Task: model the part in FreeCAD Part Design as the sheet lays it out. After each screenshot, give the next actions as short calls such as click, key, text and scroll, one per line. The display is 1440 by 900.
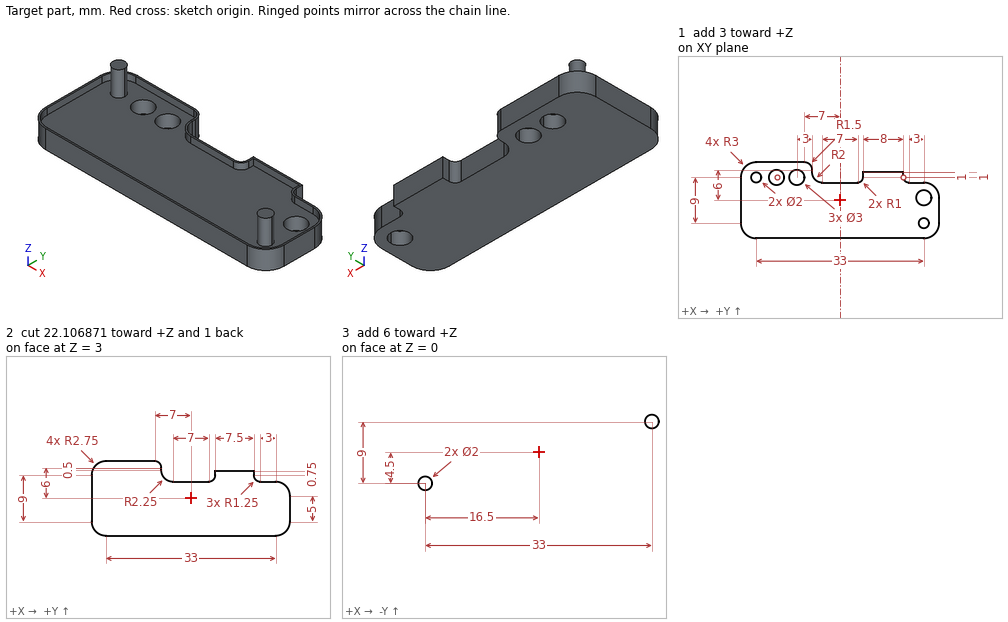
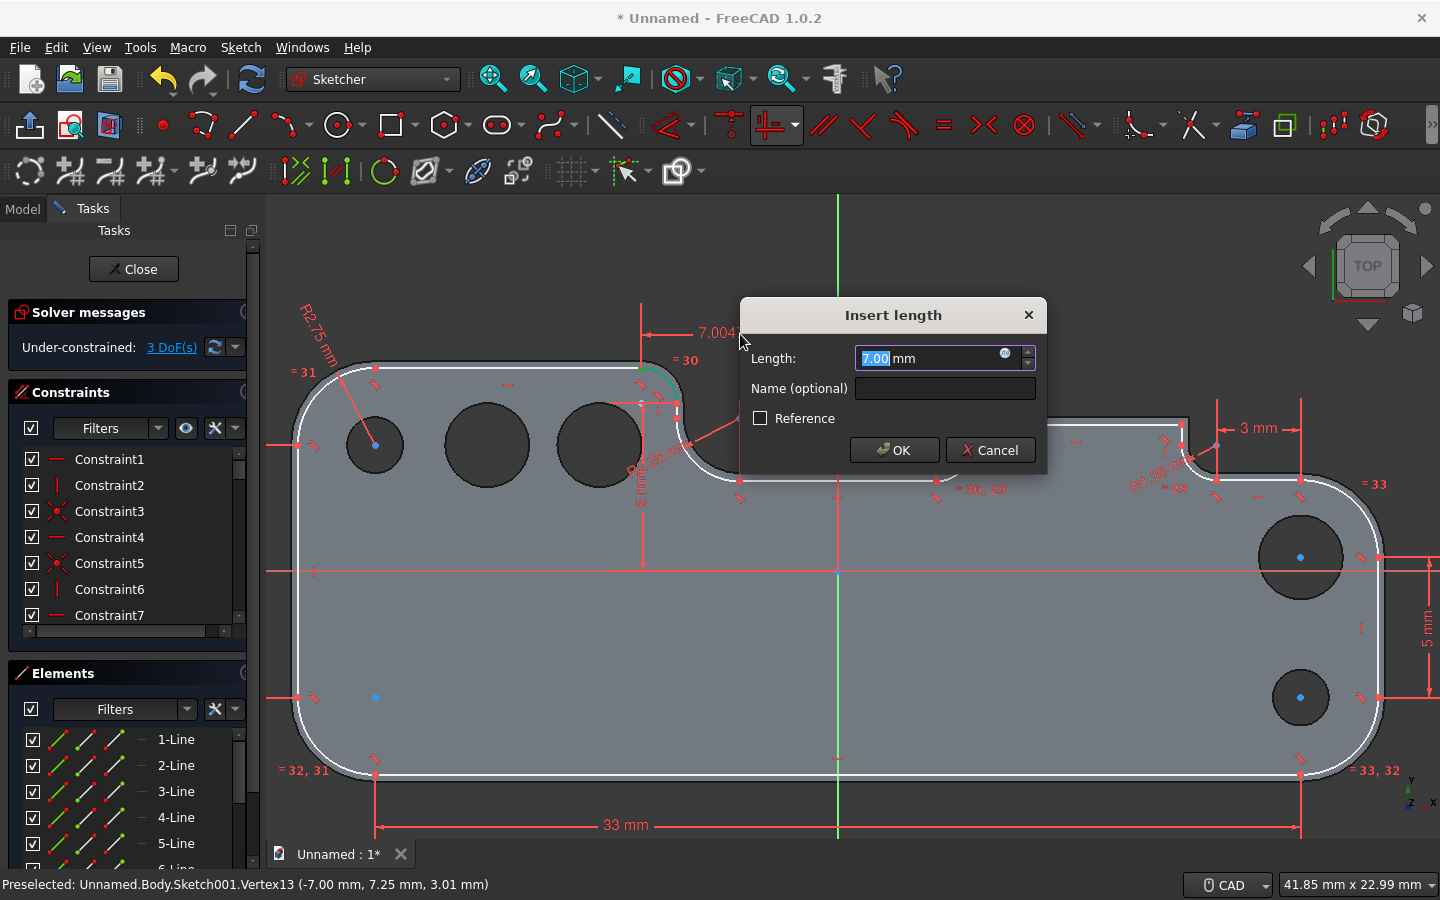
text(7)
key(Return)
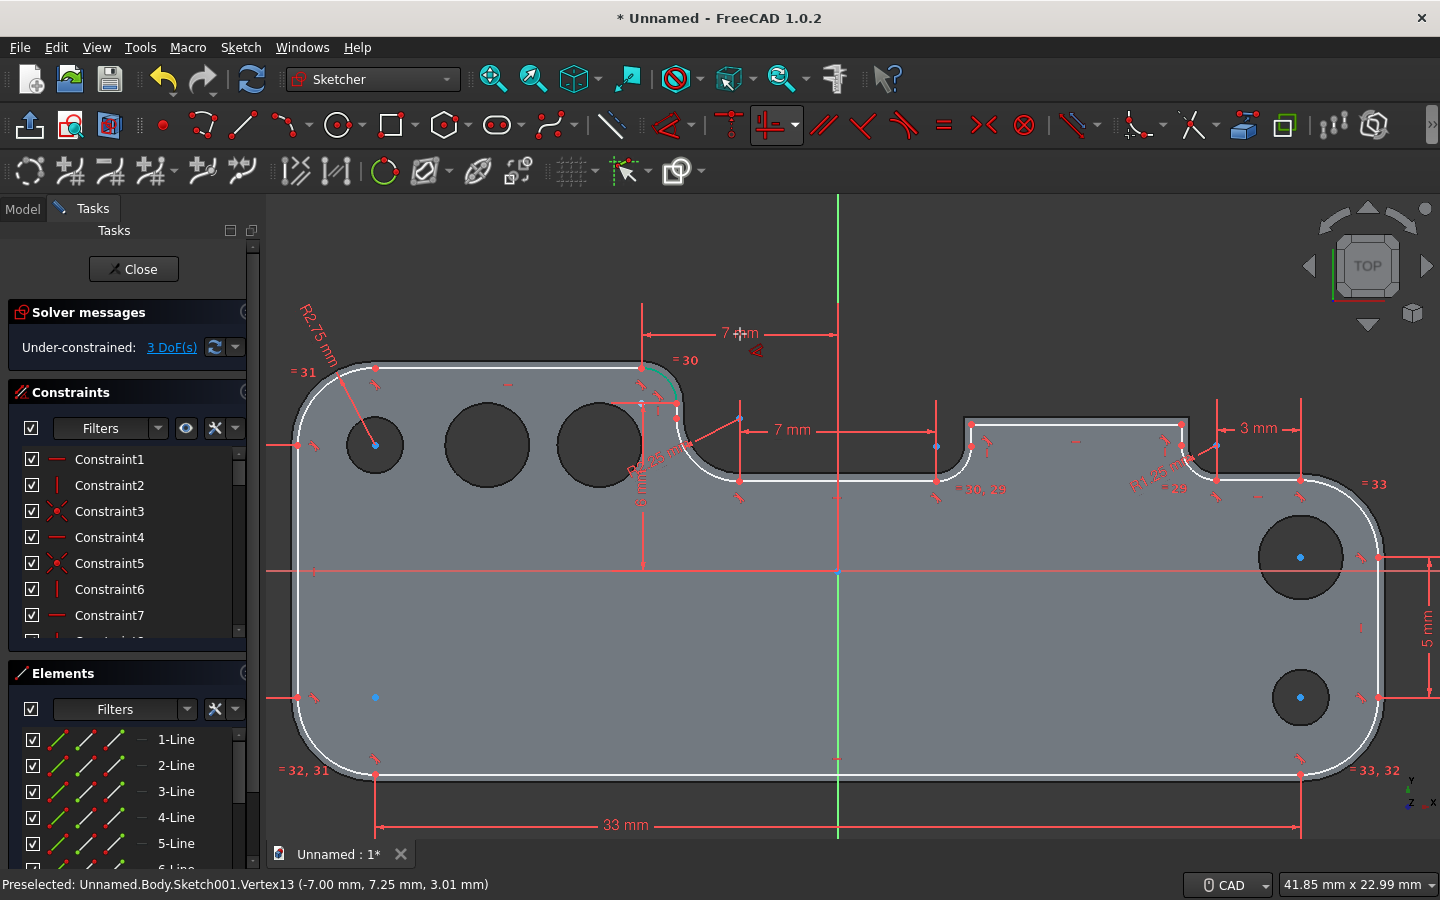
click(1119, 425)
click(1076, 391)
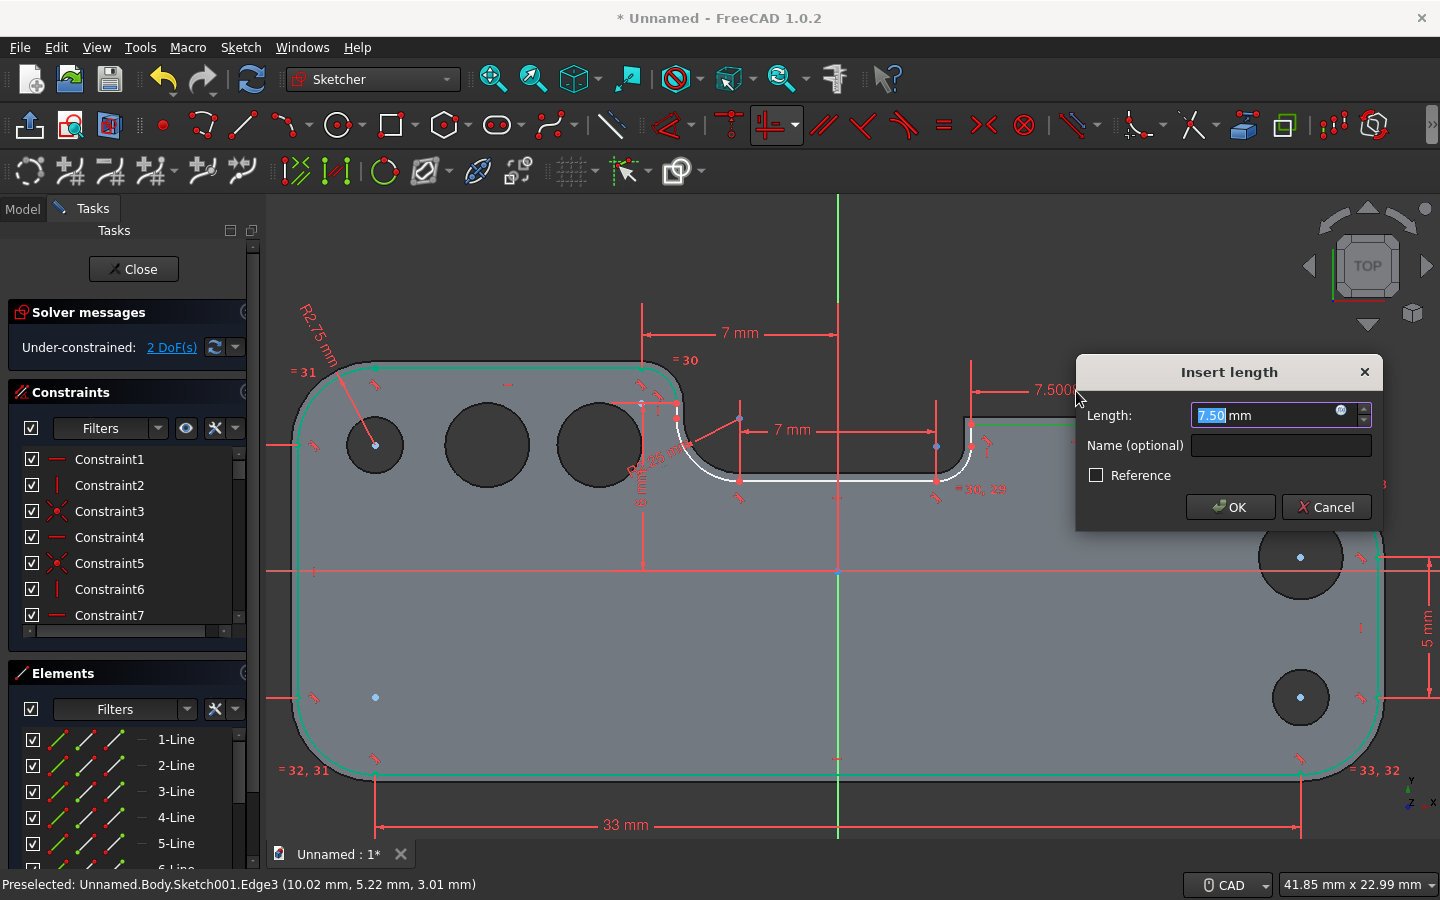
text(7.5)
key(Return)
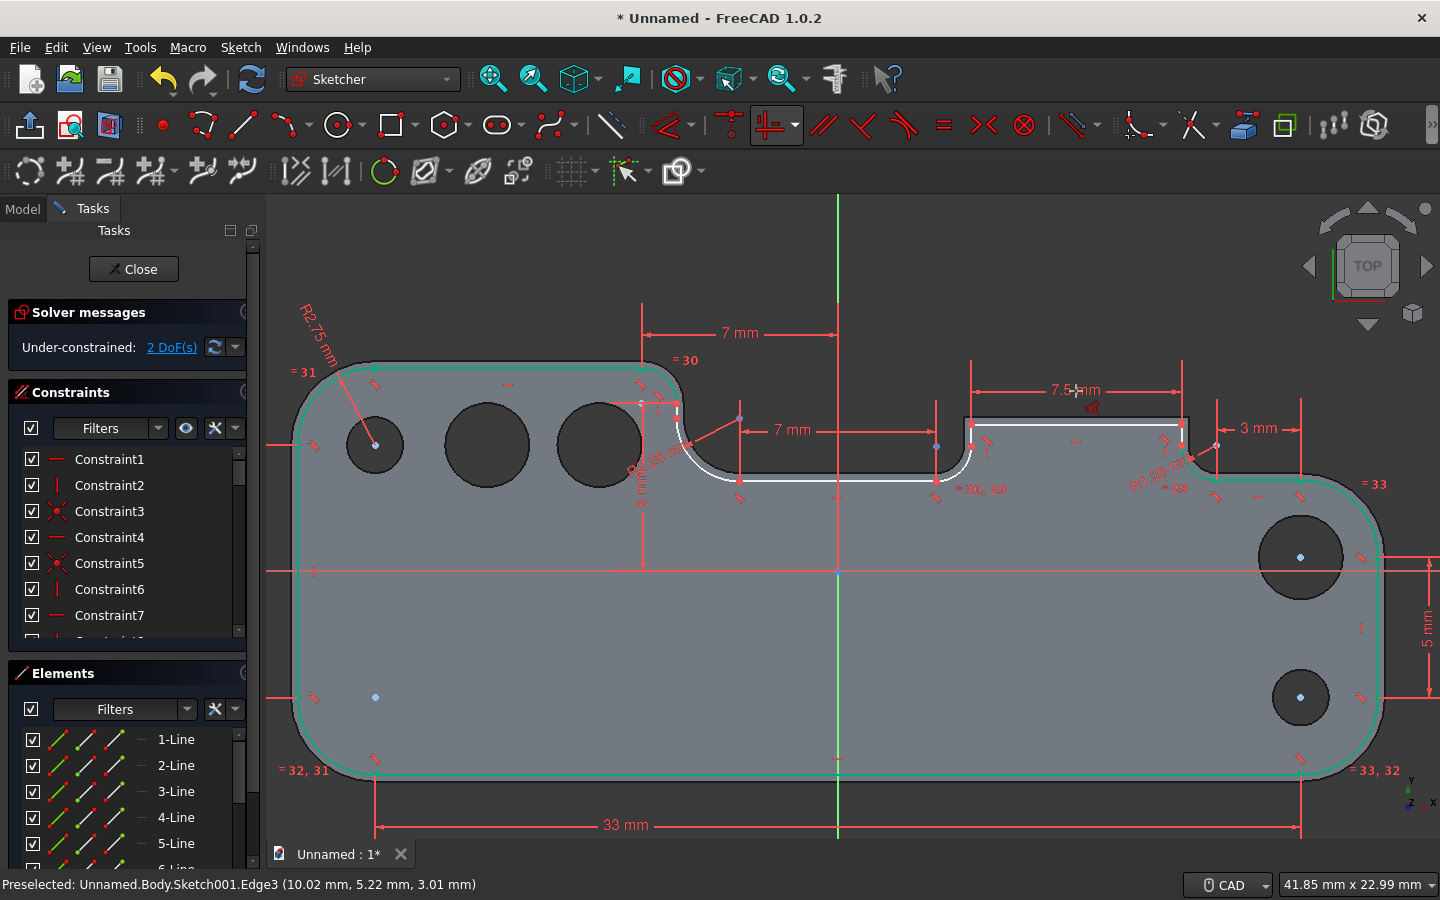
scroll(677, 411, up, 6)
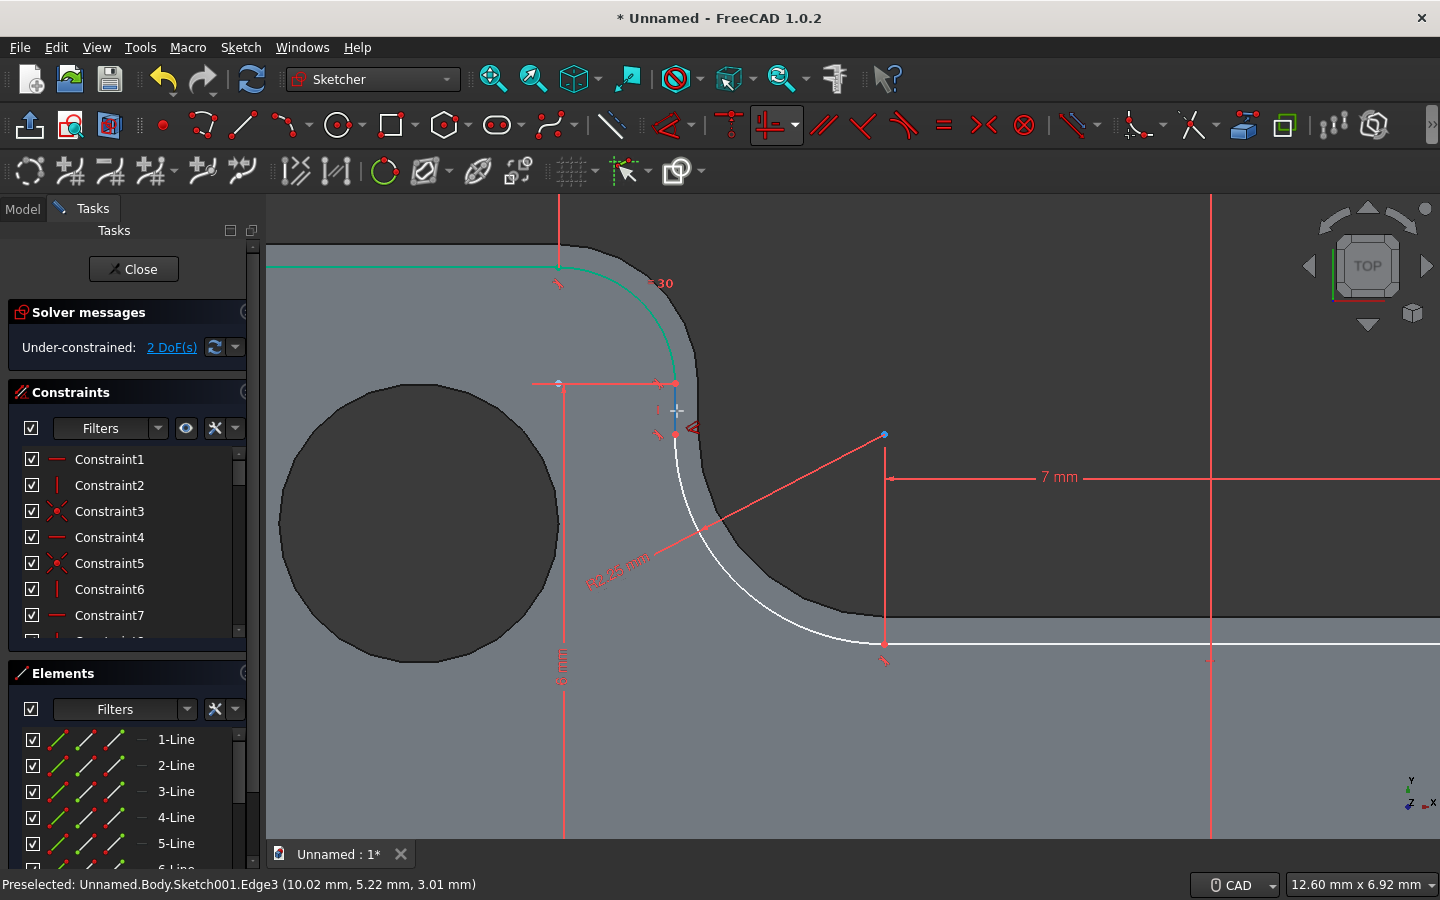
click(675, 409)
click(641, 409)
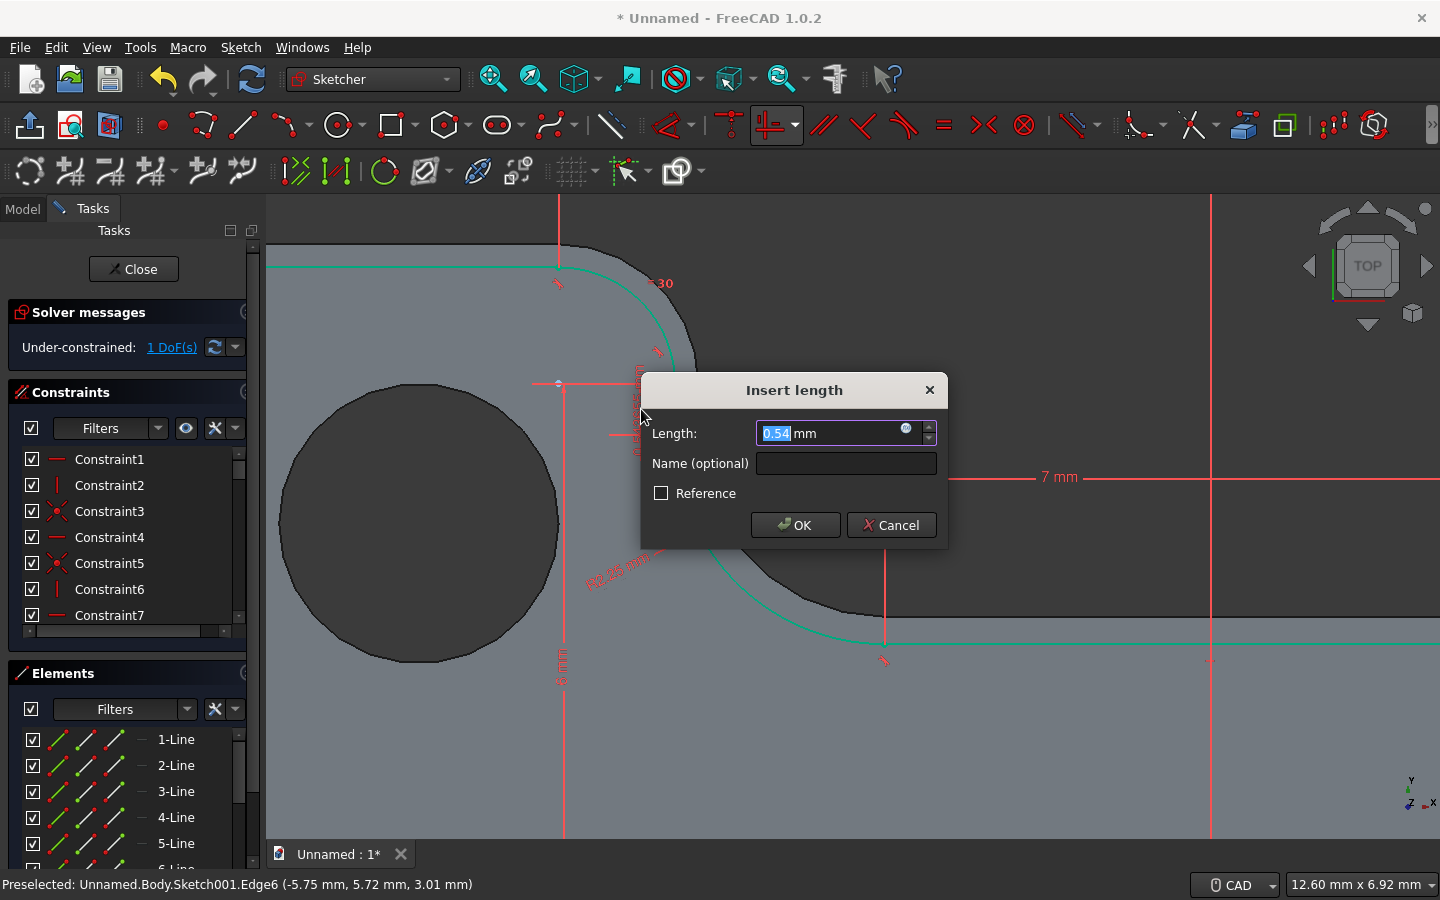
text(0.5)
key(Return)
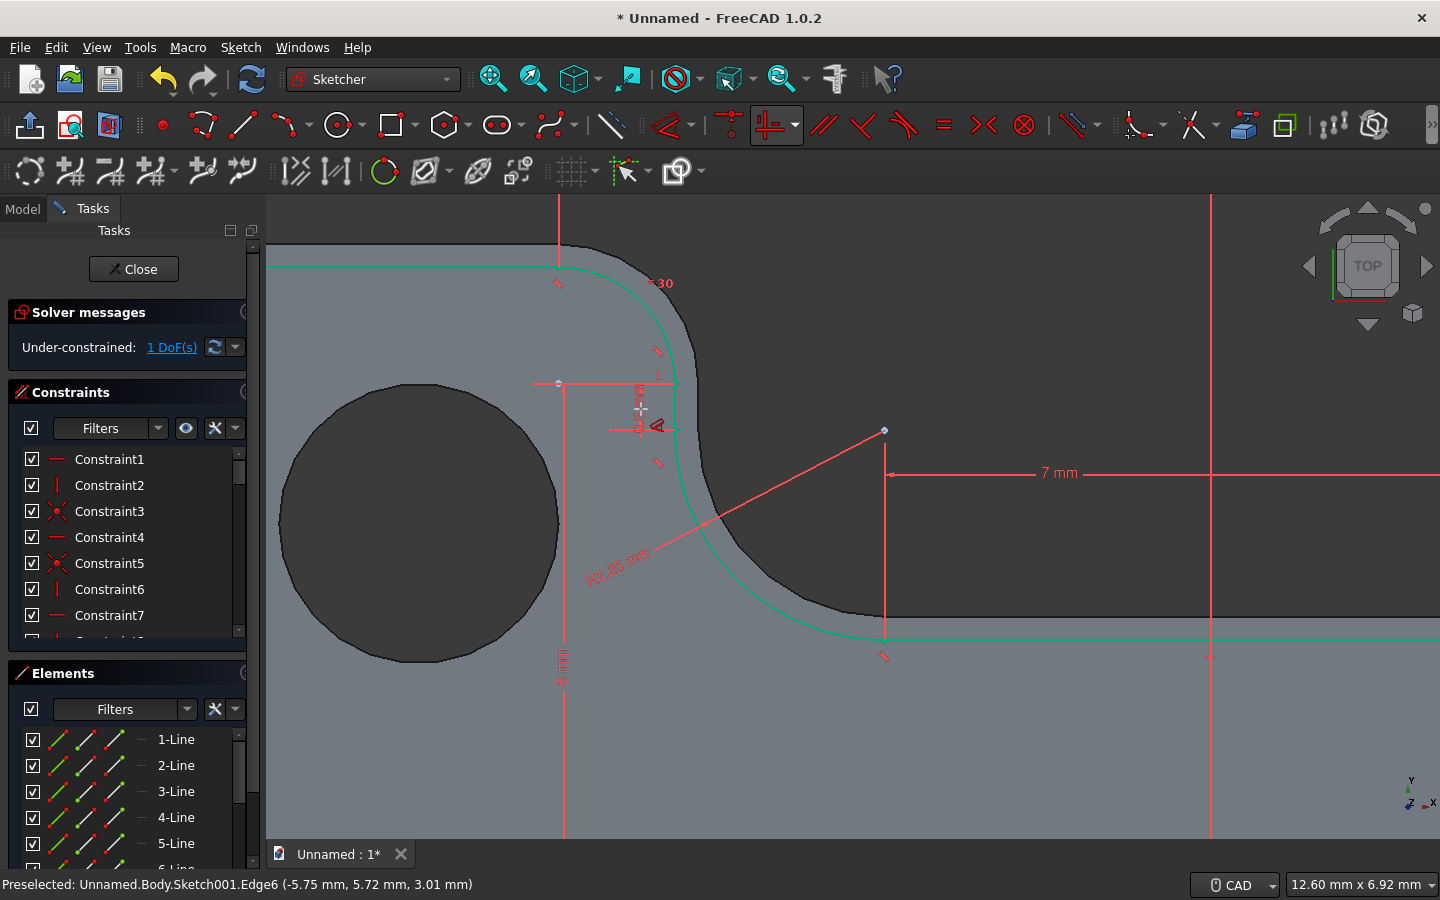
scroll(677, 409, down, 8)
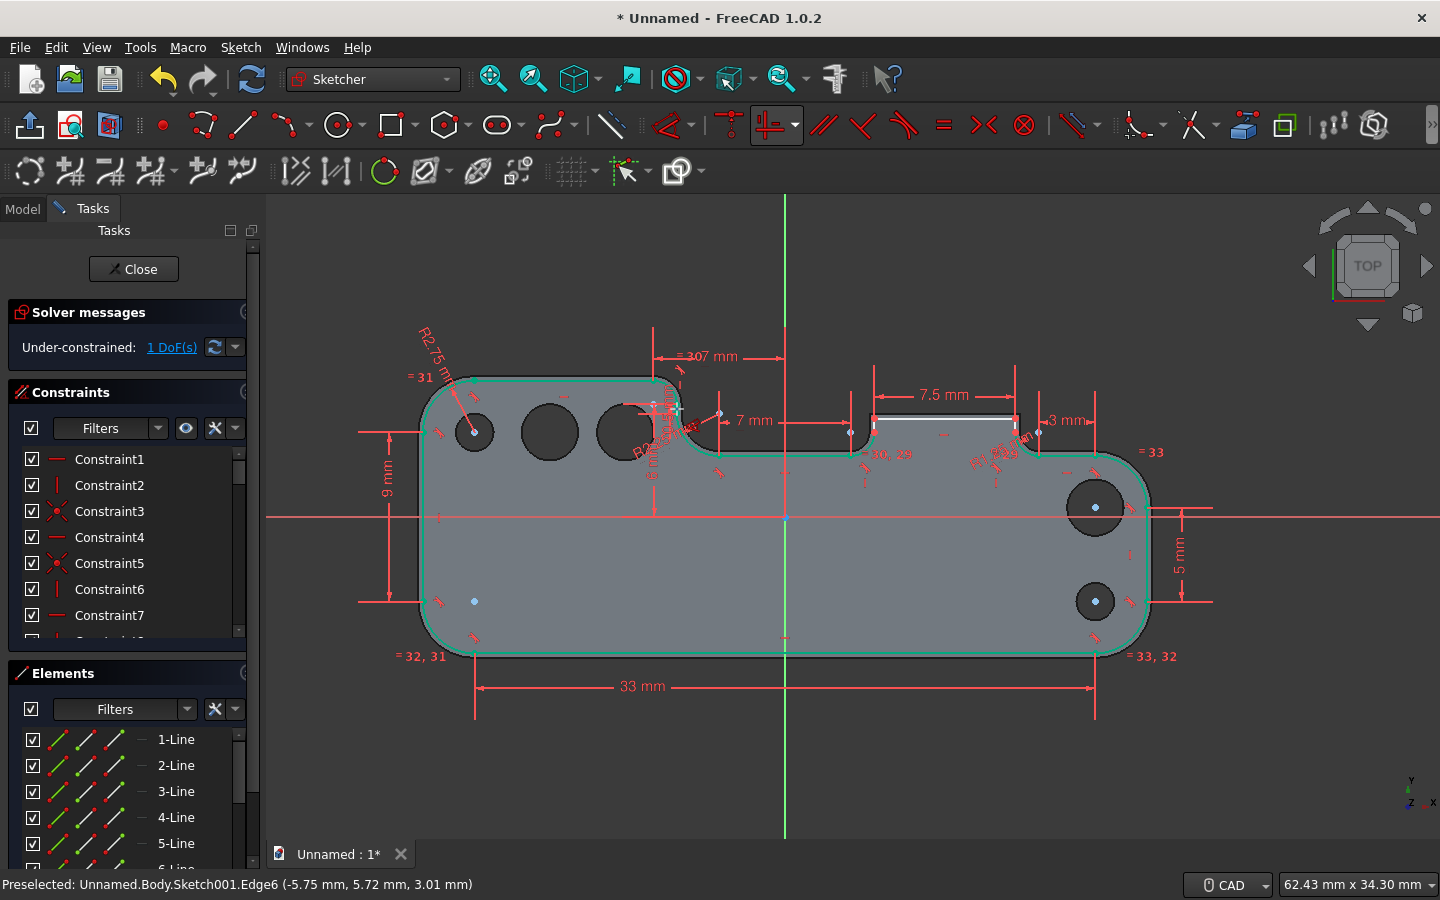
scroll(1015, 428, up, 7)